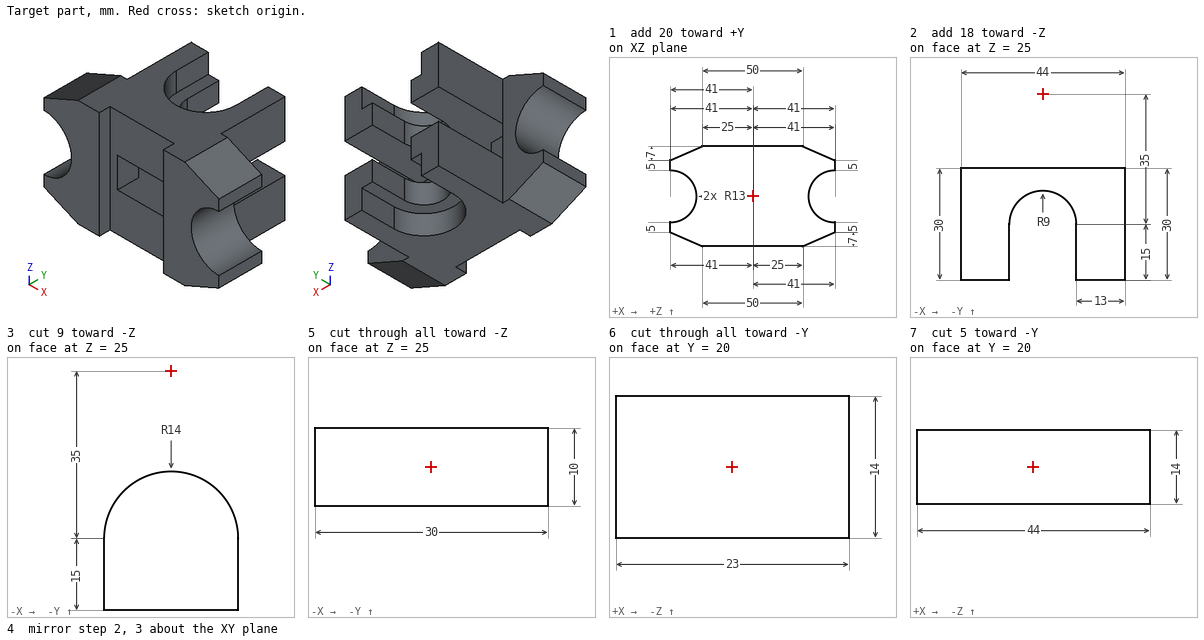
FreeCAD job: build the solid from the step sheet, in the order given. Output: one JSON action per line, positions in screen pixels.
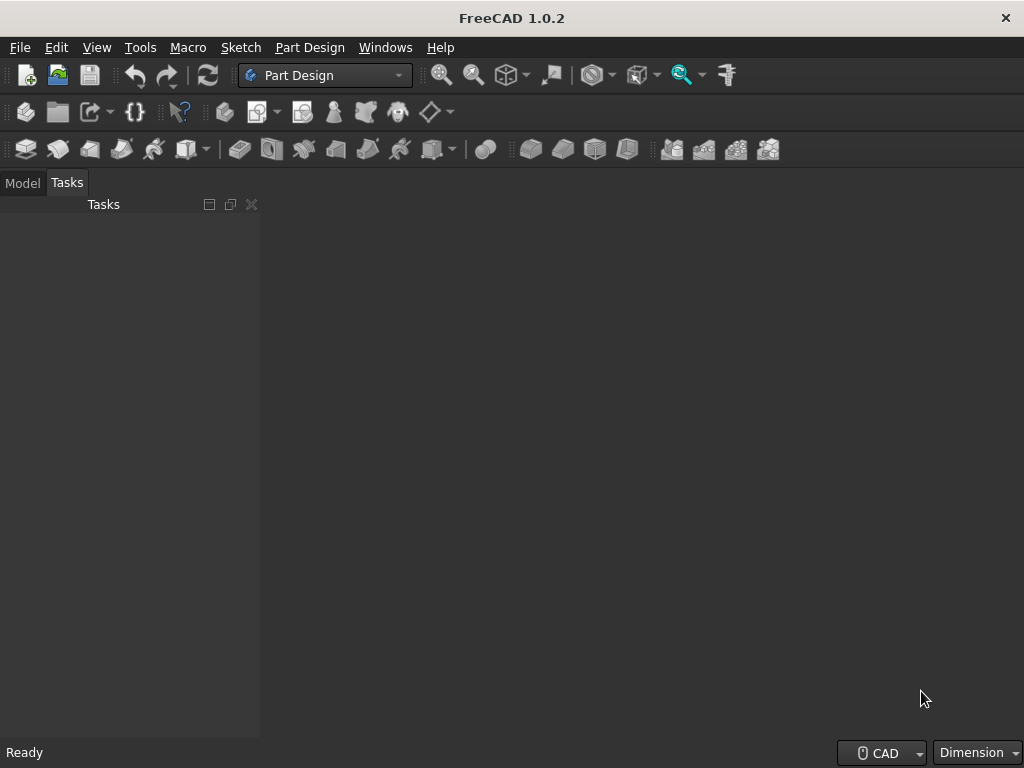
{"action": "left_click", "coordinate": [26, 76]}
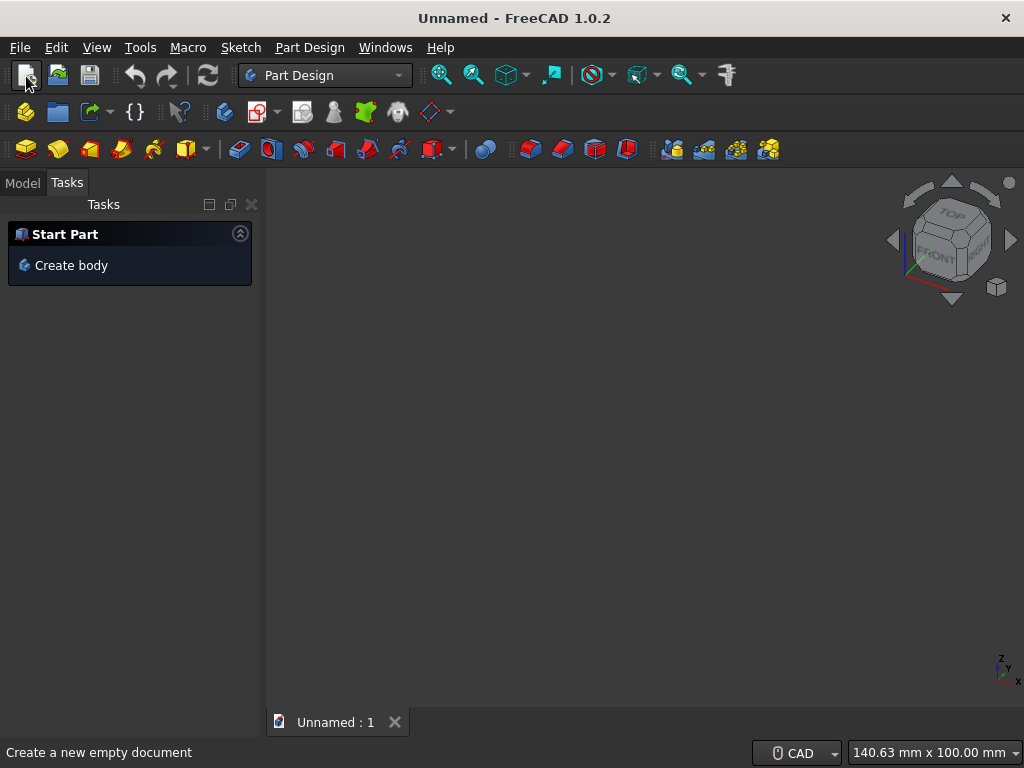
{"action": "left_click", "coordinate": [258, 112]}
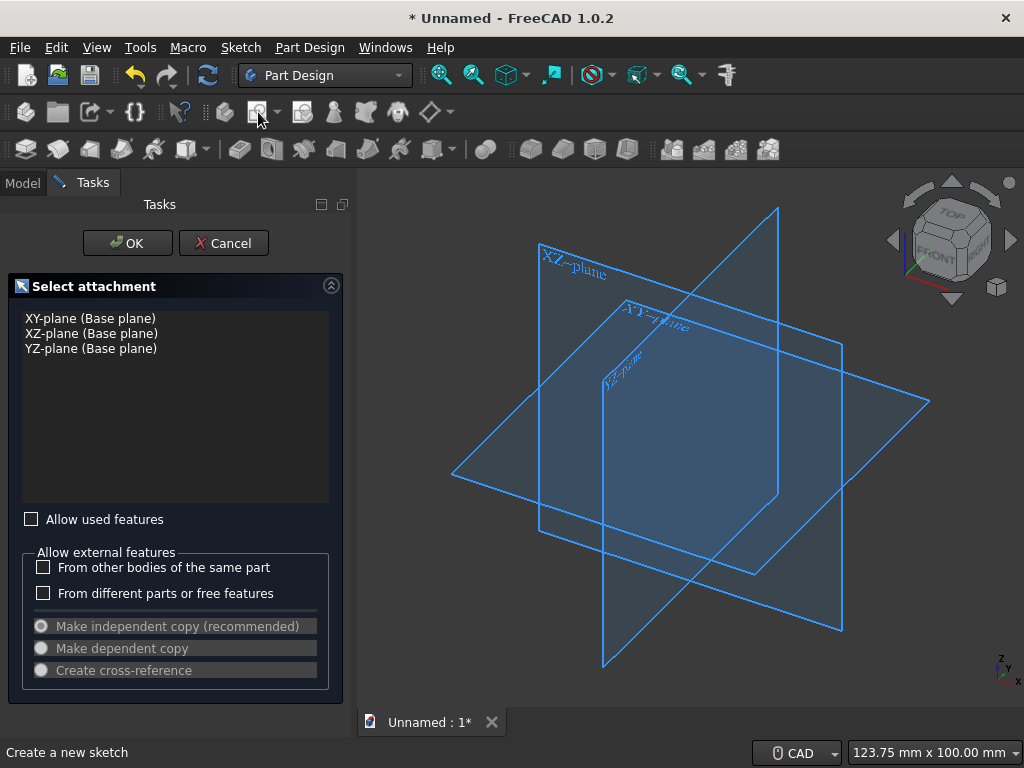
{"action": "left_click", "coordinate": [82, 334]}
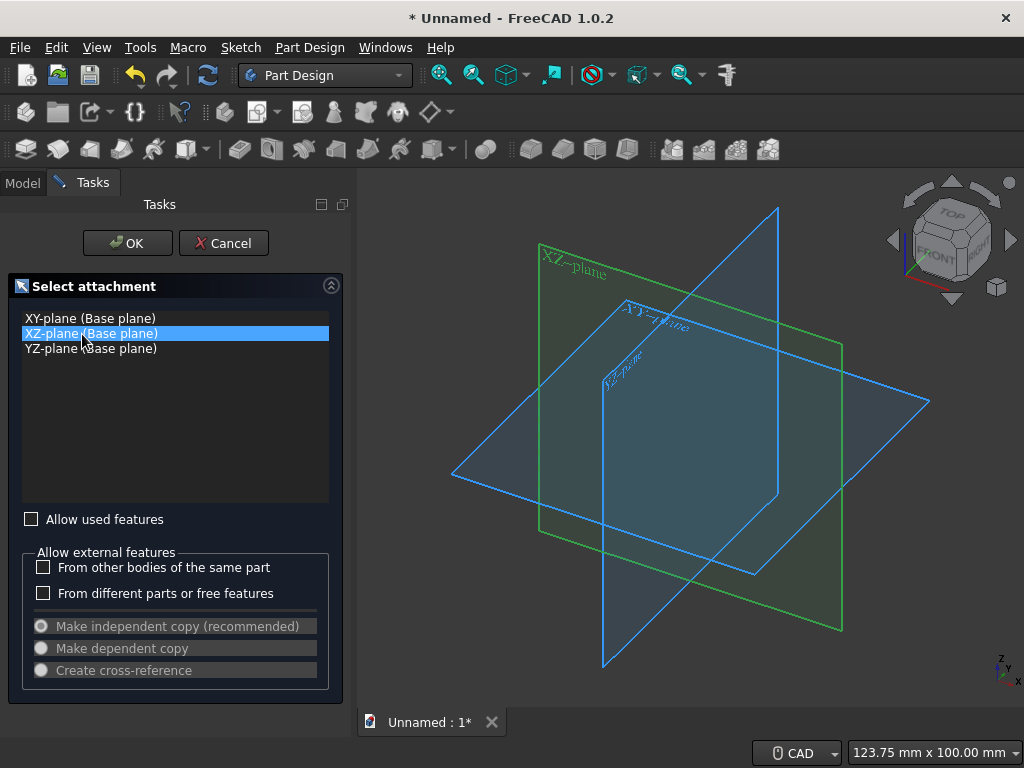
{"action": "left_click", "coordinate": [128, 243]}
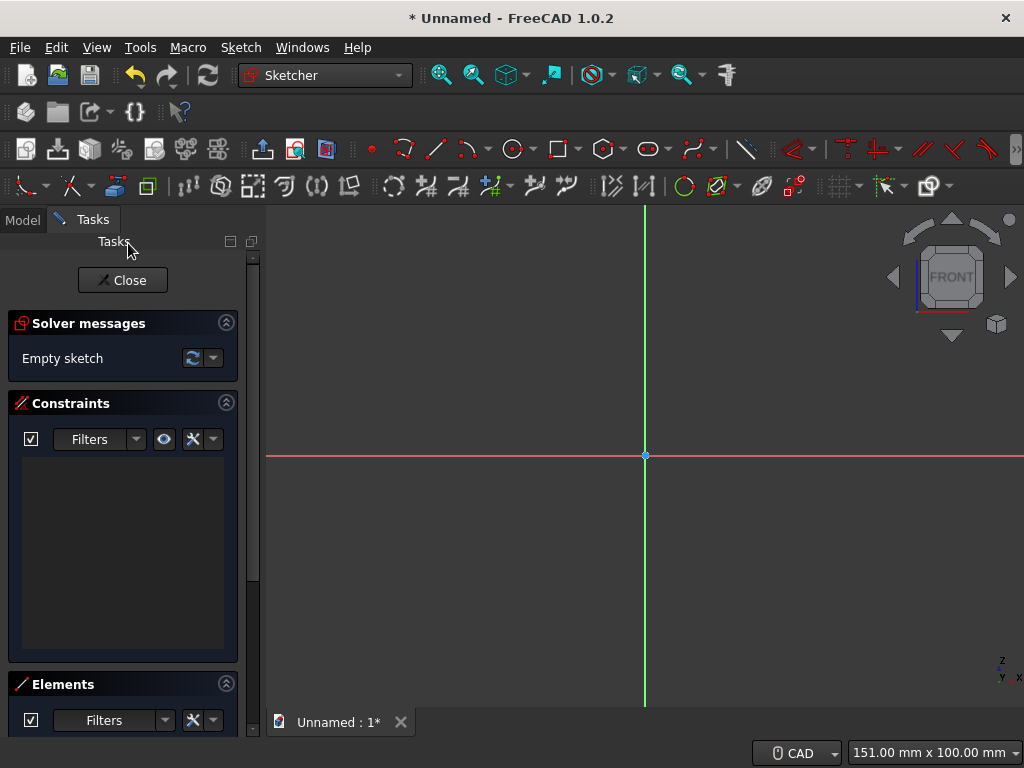
{"action": "scroll", "coordinate": [294, 456], "scroll_direction": "down", "scroll_amount": 1}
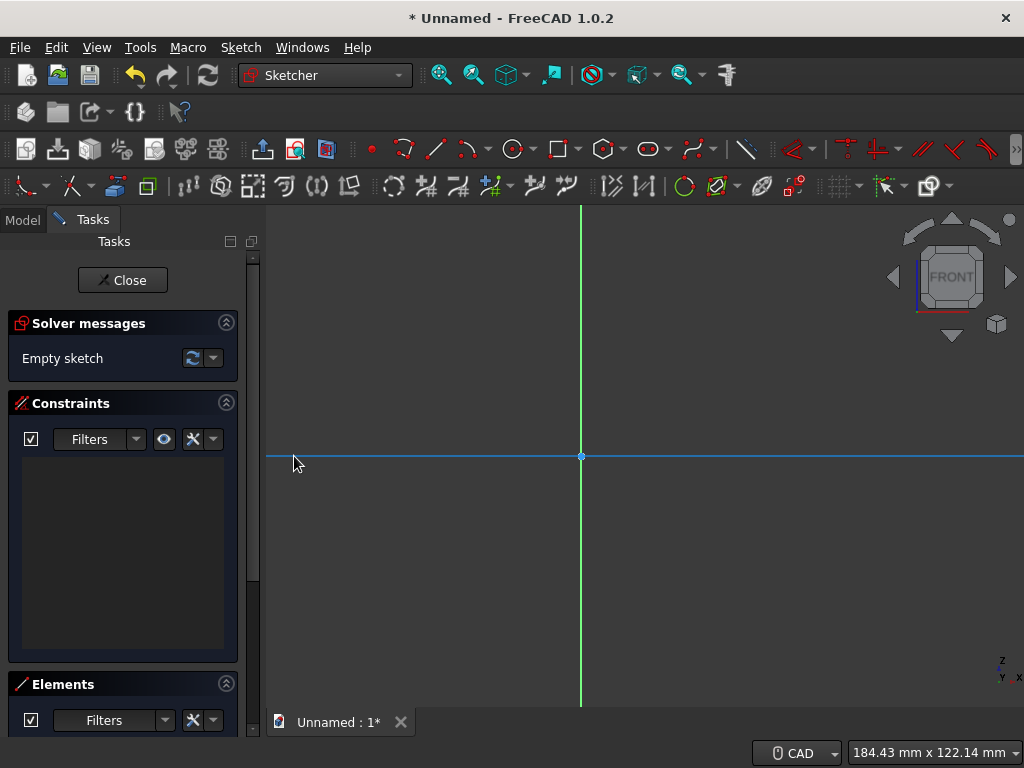
{"action": "left_click", "coordinate": [404, 150]}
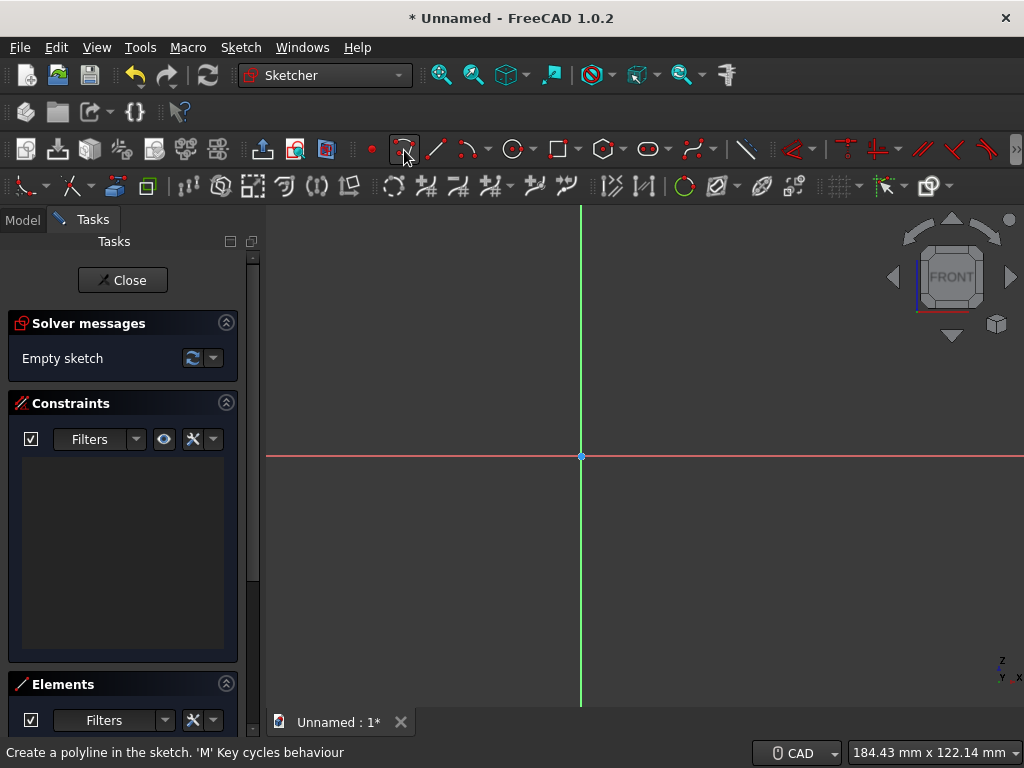
{"action": "left_click", "coordinate": [413, 403]}
{"action": "left_click", "coordinate": [413, 382]}
{"action": "left_click", "coordinate": [479, 353]}
{"action": "left_click", "coordinate": [684, 353]}
{"action": "left_click", "coordinate": [750, 382]}
{"action": "left_click", "coordinate": [750, 403]}
{"action": "right_click", "coordinate": [750, 403]}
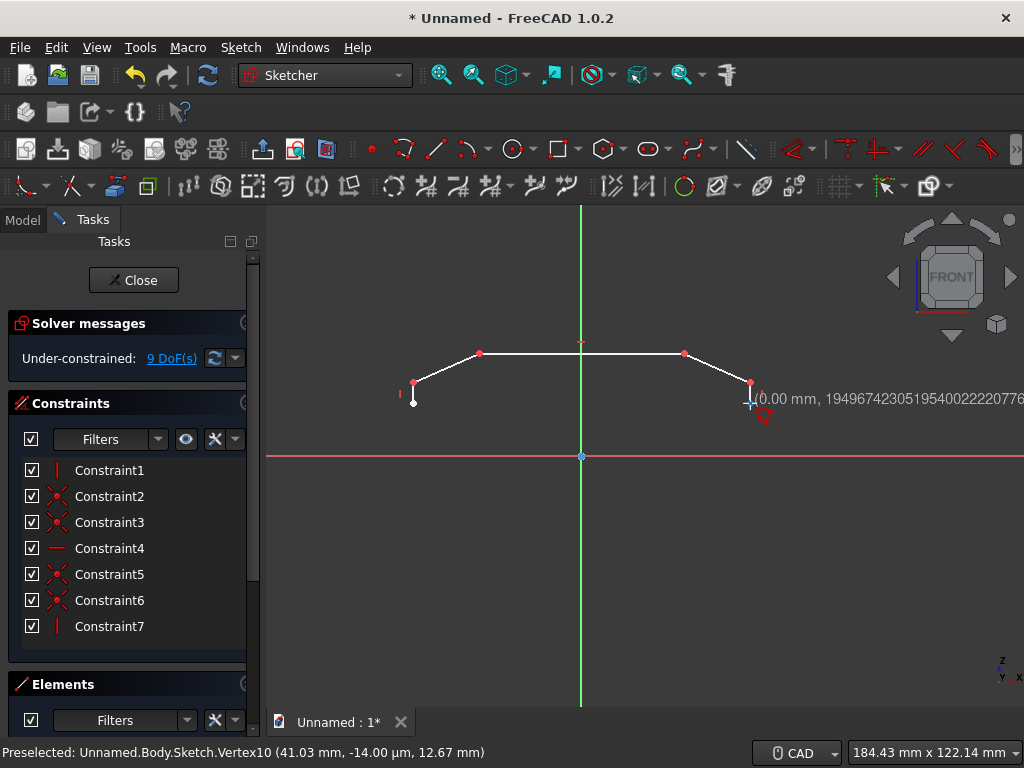
{"action": "left_click", "coordinate": [750, 510]}
{"action": "left_click", "coordinate": [750, 530]}
{"action": "left_click", "coordinate": [684, 559]}
{"action": "left_click", "coordinate": [479, 559]}
{"action": "left_click", "coordinate": [413, 530]}
{"action": "left_click", "coordinate": [413, 510]}
{"action": "right_click", "coordinate": [413, 510]}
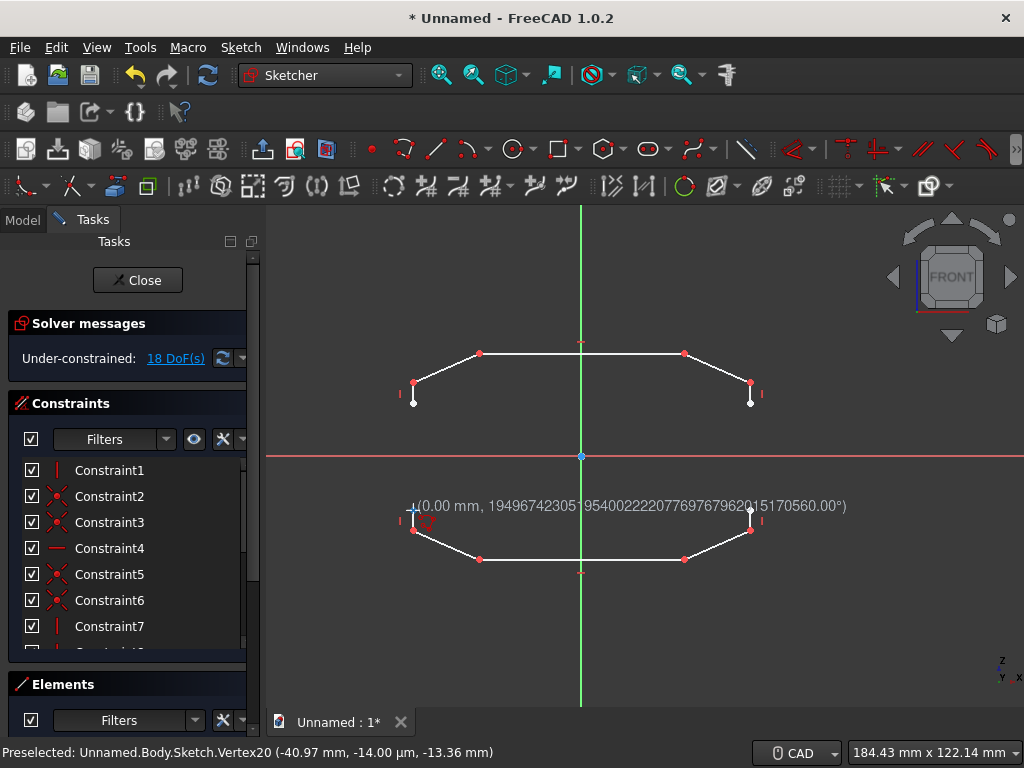
{"action": "left_click", "coordinate": [490, 150]}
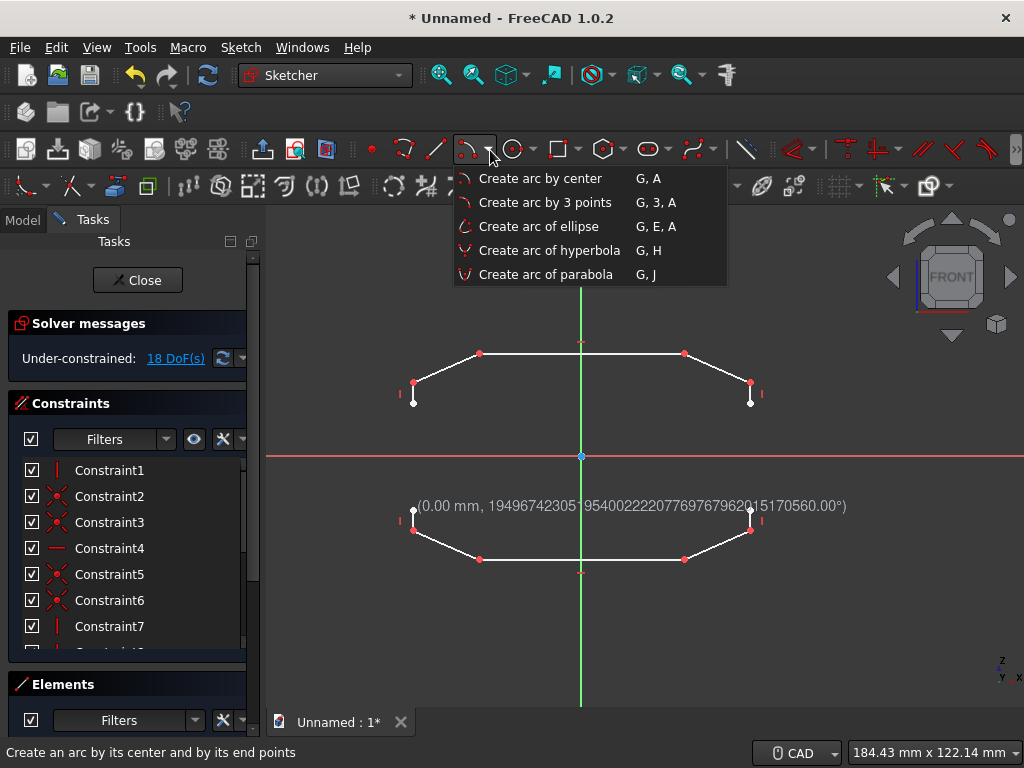
{"action": "left_click", "coordinate": [590, 202]}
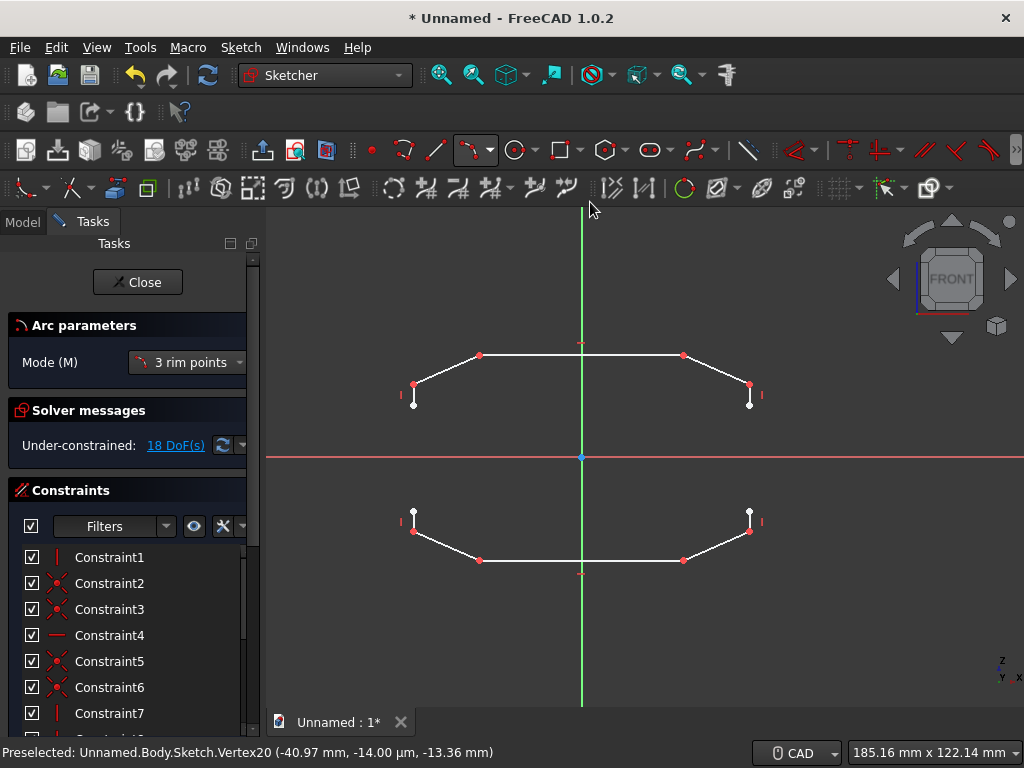
{"action": "scroll", "coordinate": [749, 404], "scroll_direction": "up", "scroll_amount": 3}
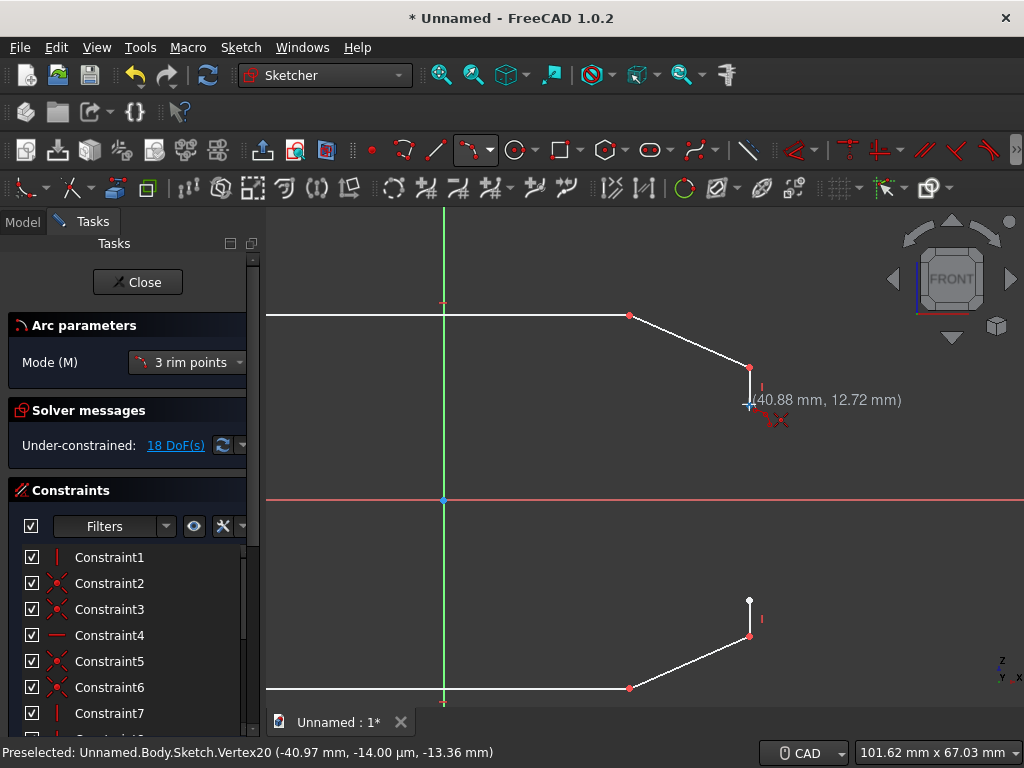
{"action": "left_click", "coordinate": [750, 406]}
{"action": "left_click", "coordinate": [750, 600]}
{"action": "left_click", "coordinate": [657, 470]}